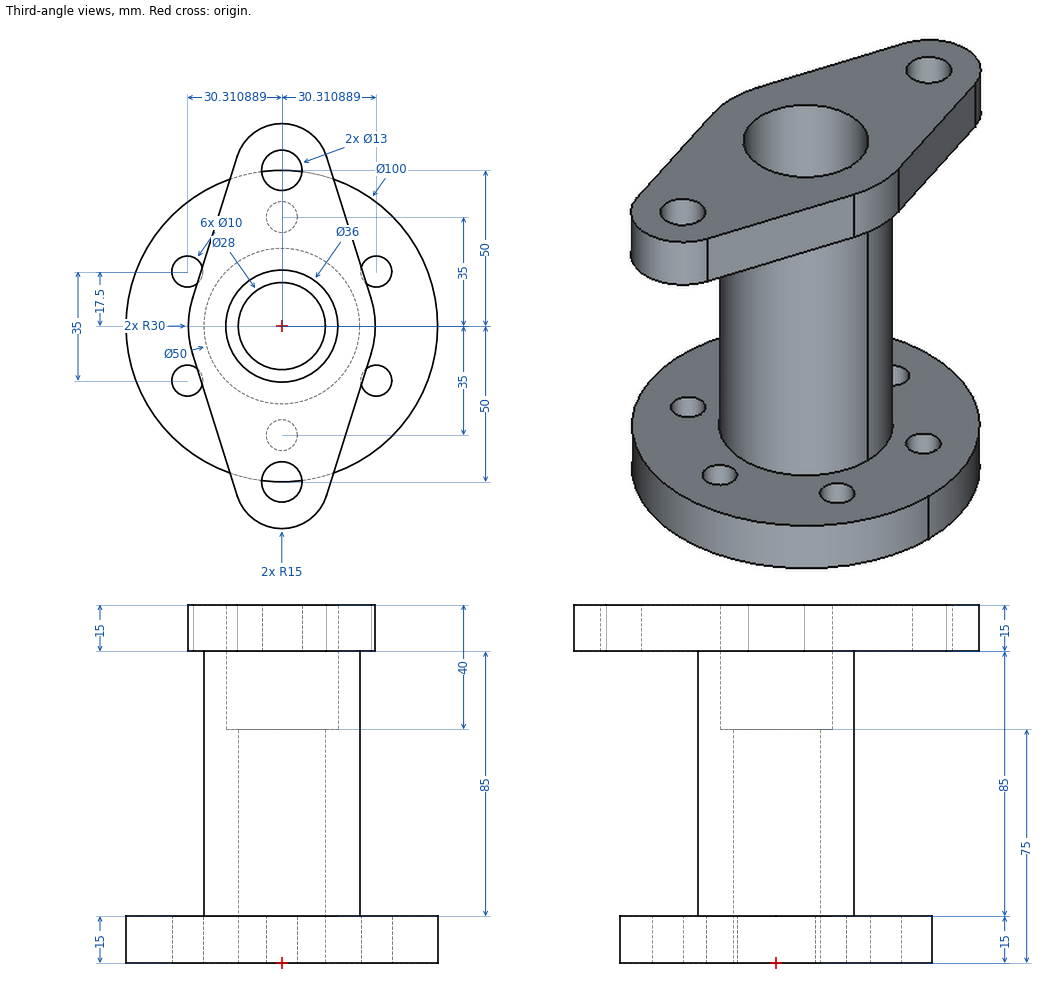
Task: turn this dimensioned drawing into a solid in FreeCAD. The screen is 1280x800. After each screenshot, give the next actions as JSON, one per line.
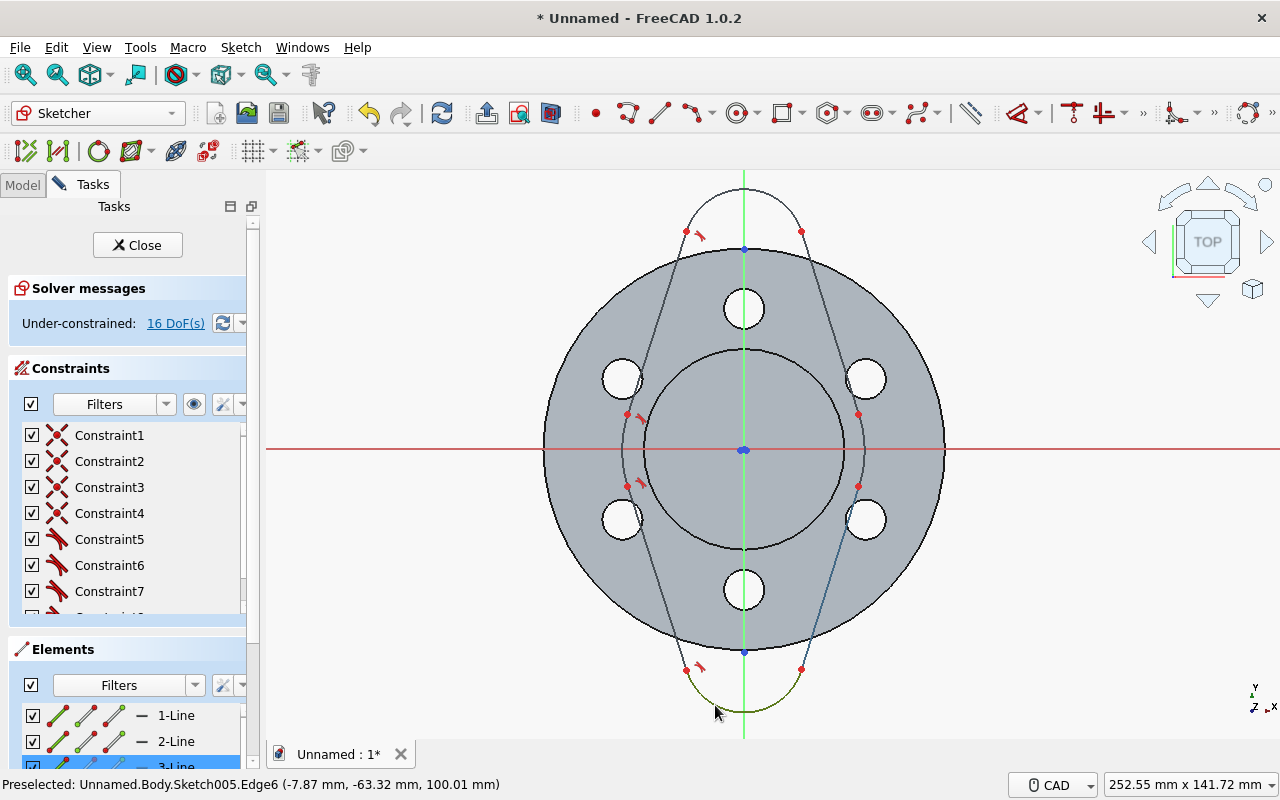
{"action": "key", "text": "t"}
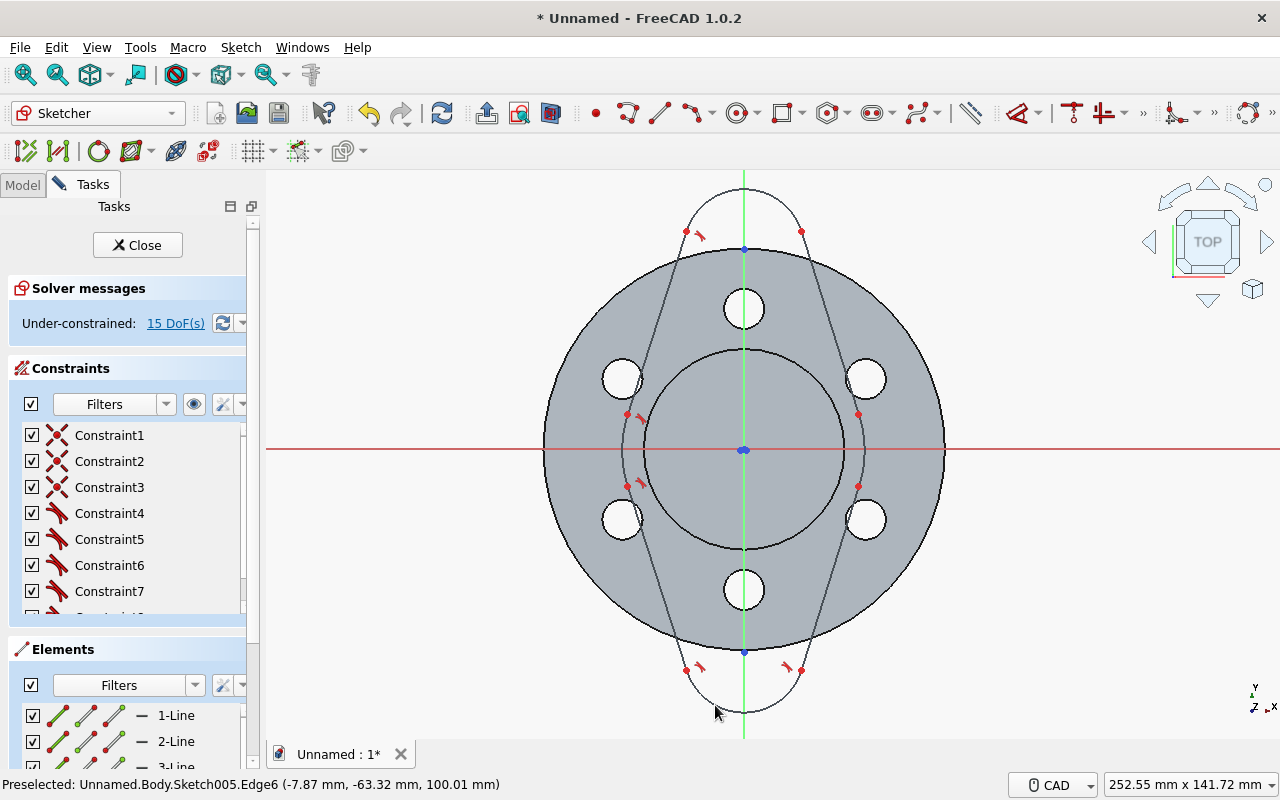
{"action": "left_click", "coordinate": [819, 615]}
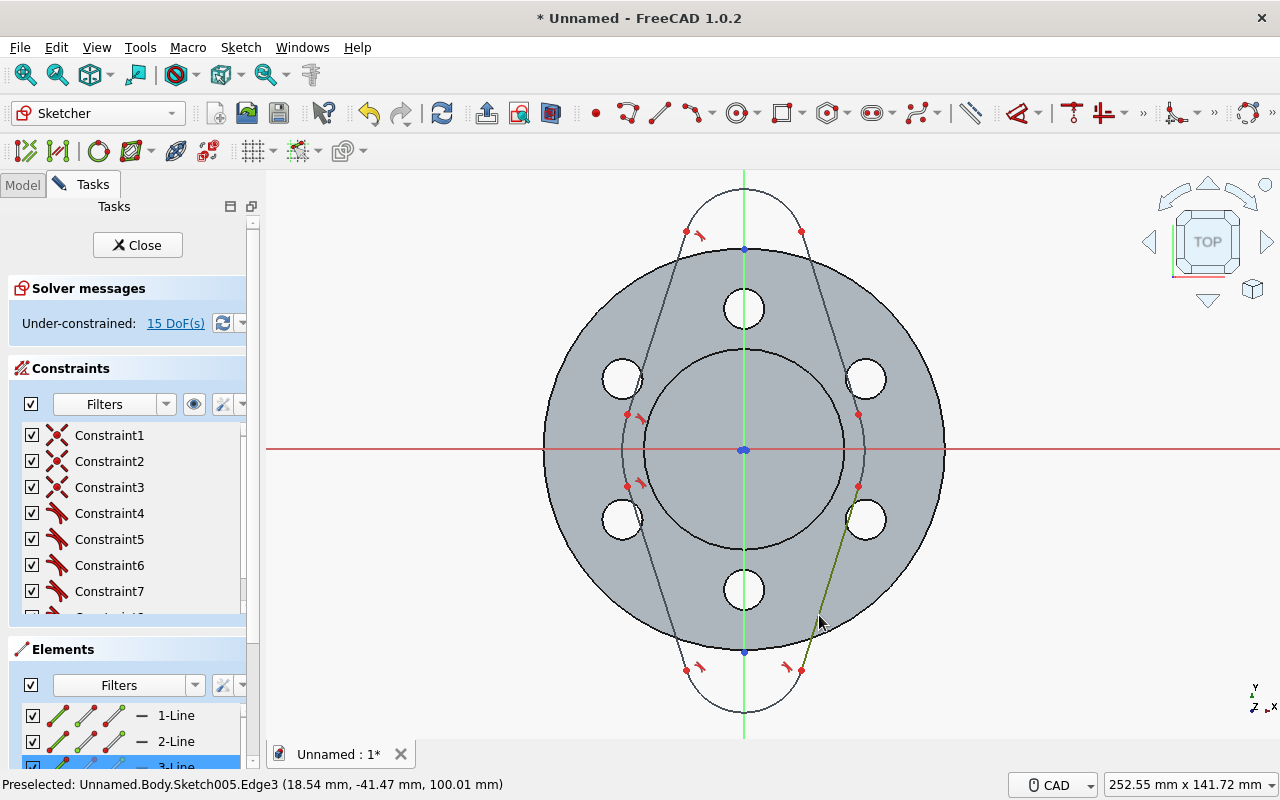
{"action": "left_click", "coordinate": [864, 465]}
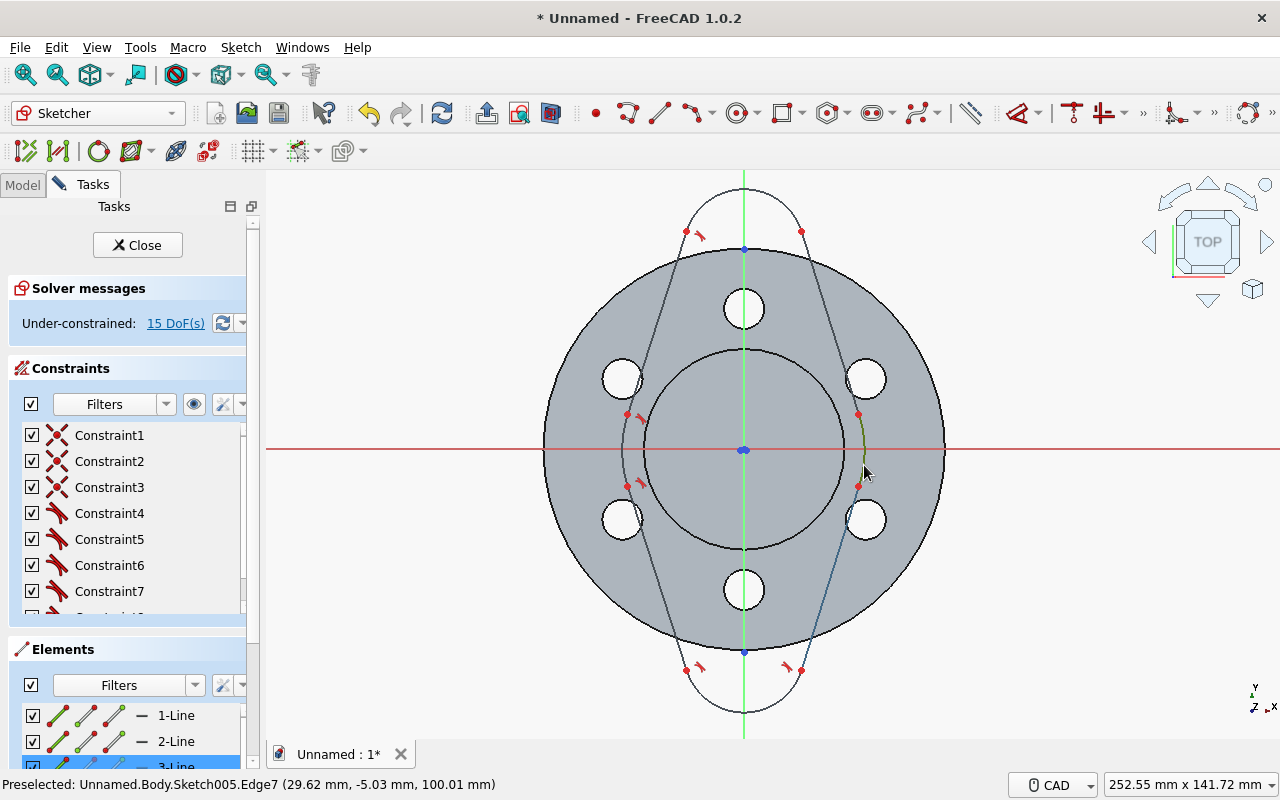
{"action": "key", "text": "t"}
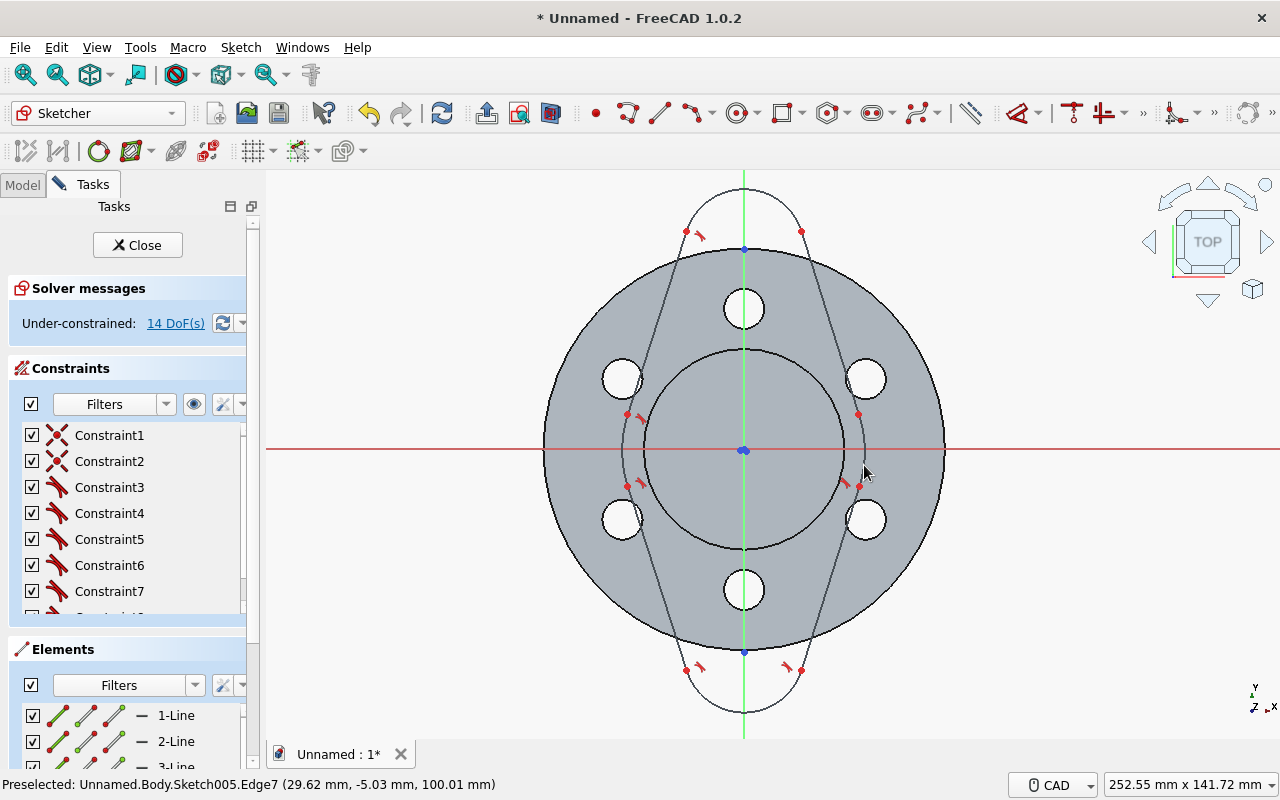
{"action": "left_click", "coordinate": [842, 360]}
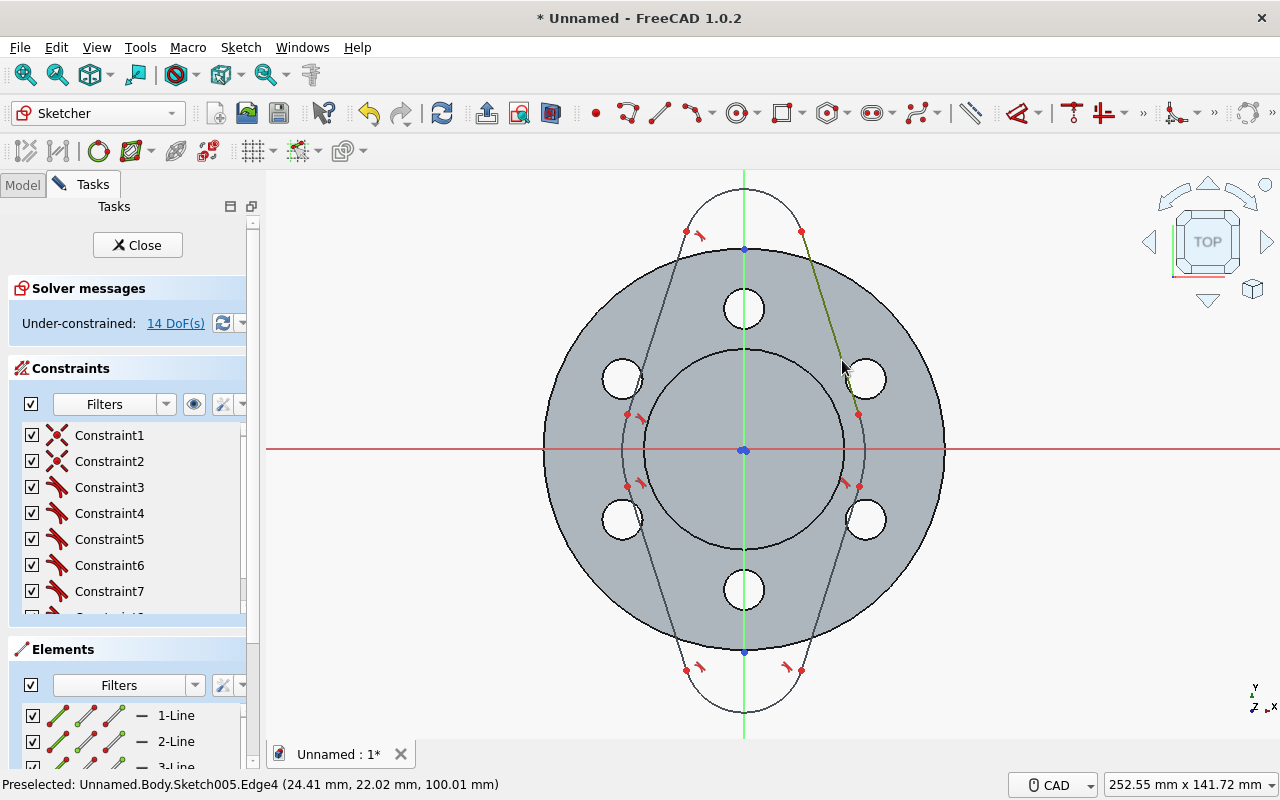
{"action": "left_click", "coordinate": [864, 465]}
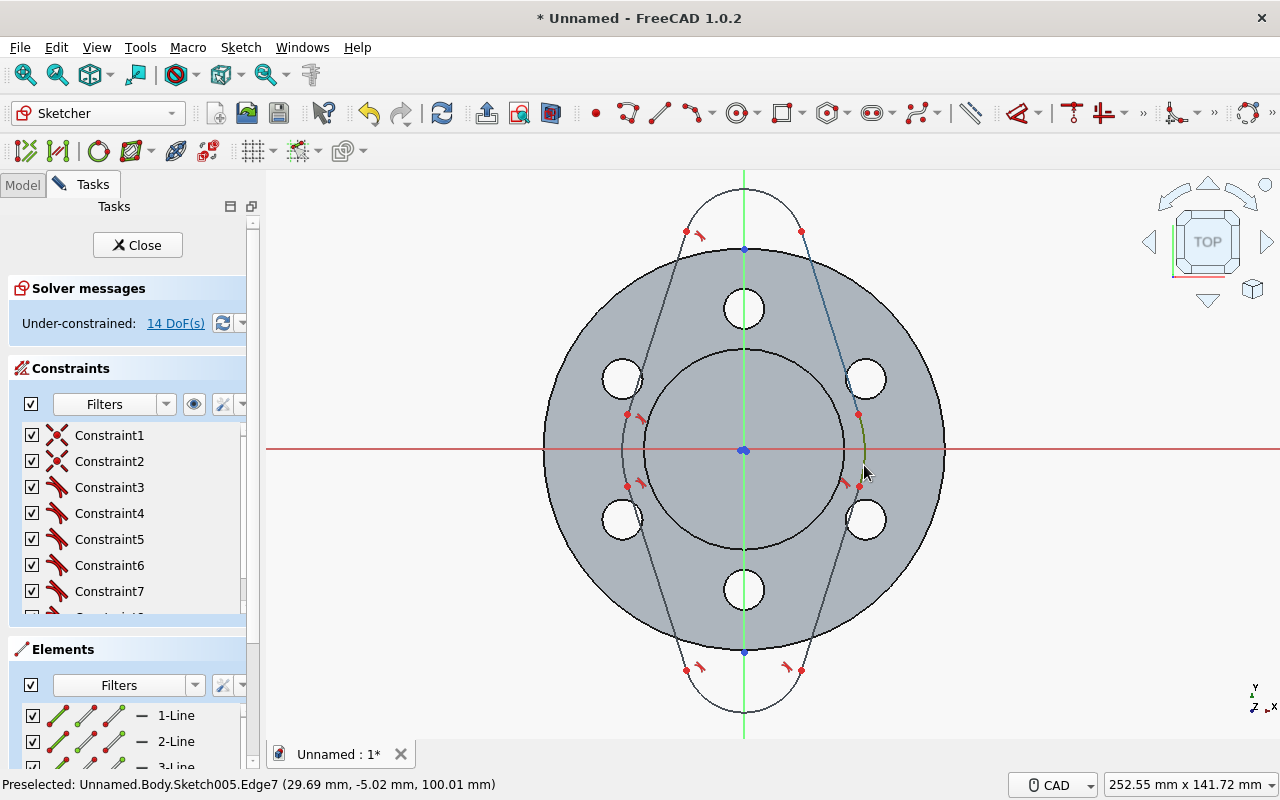
{"action": "key", "text": "t"}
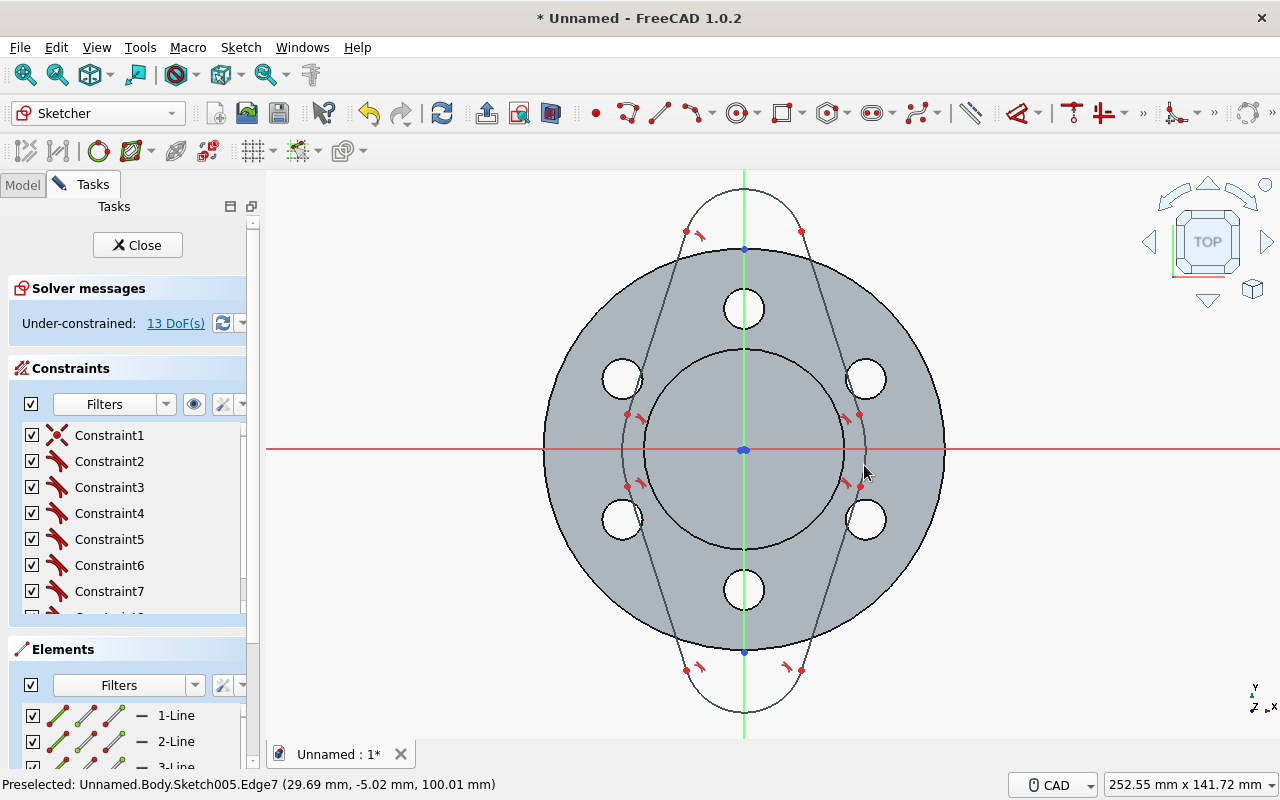
{"action": "left_click", "coordinate": [842, 360]}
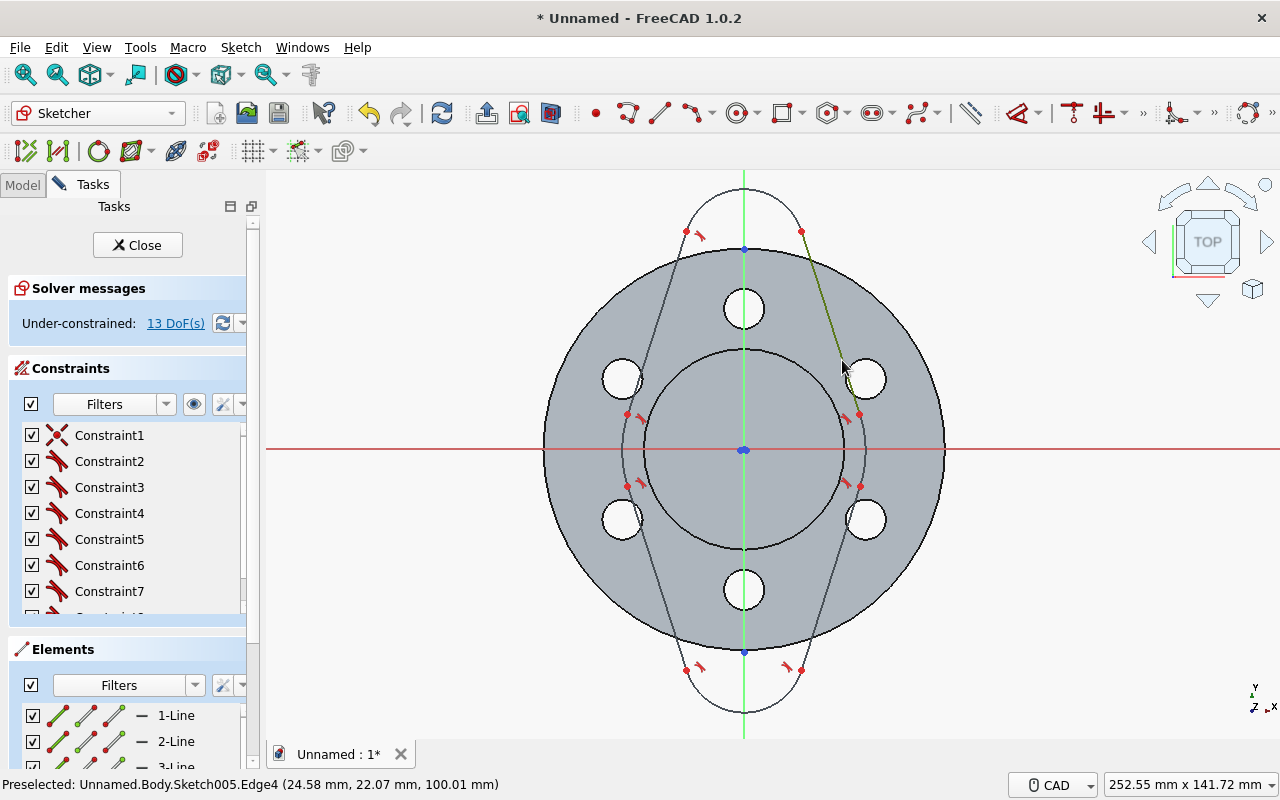
{"action": "left_click", "coordinate": [786, 206]}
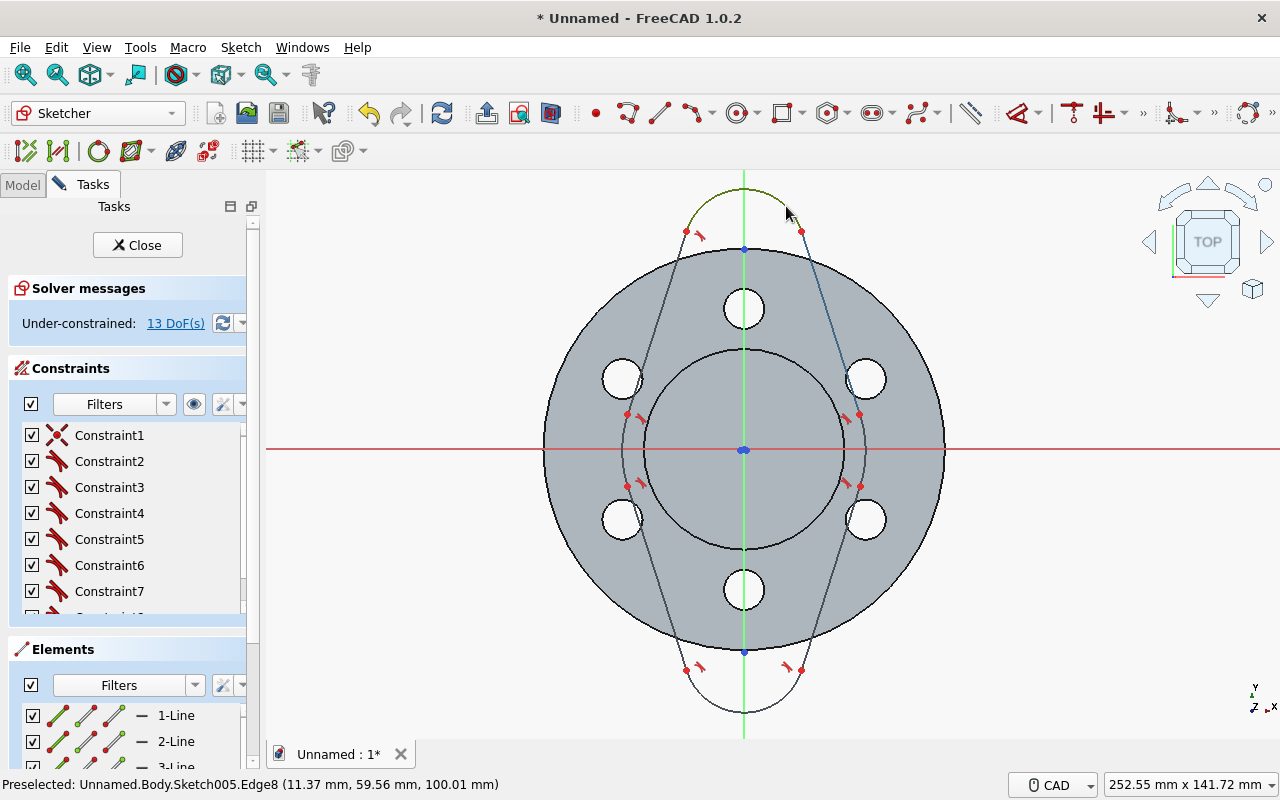
{"action": "key", "text": "t"}